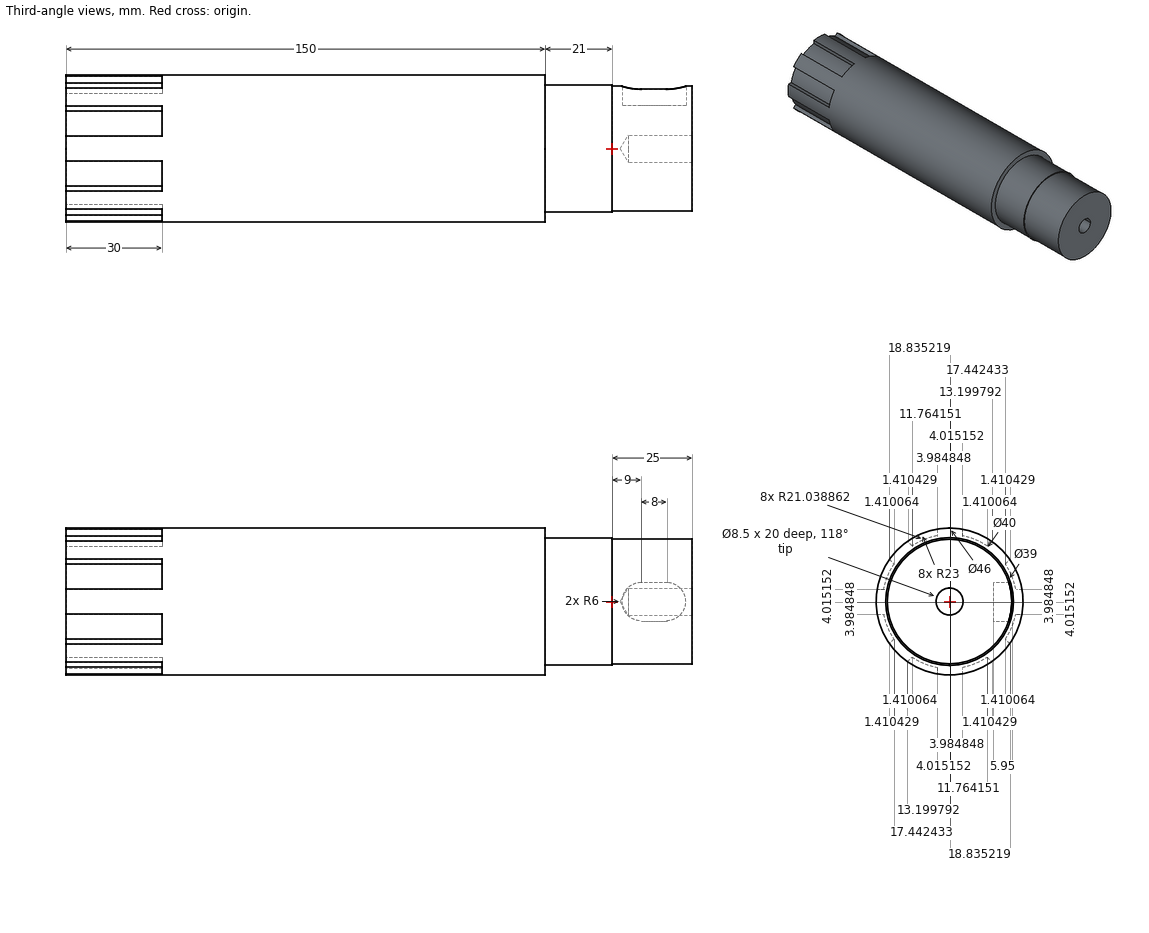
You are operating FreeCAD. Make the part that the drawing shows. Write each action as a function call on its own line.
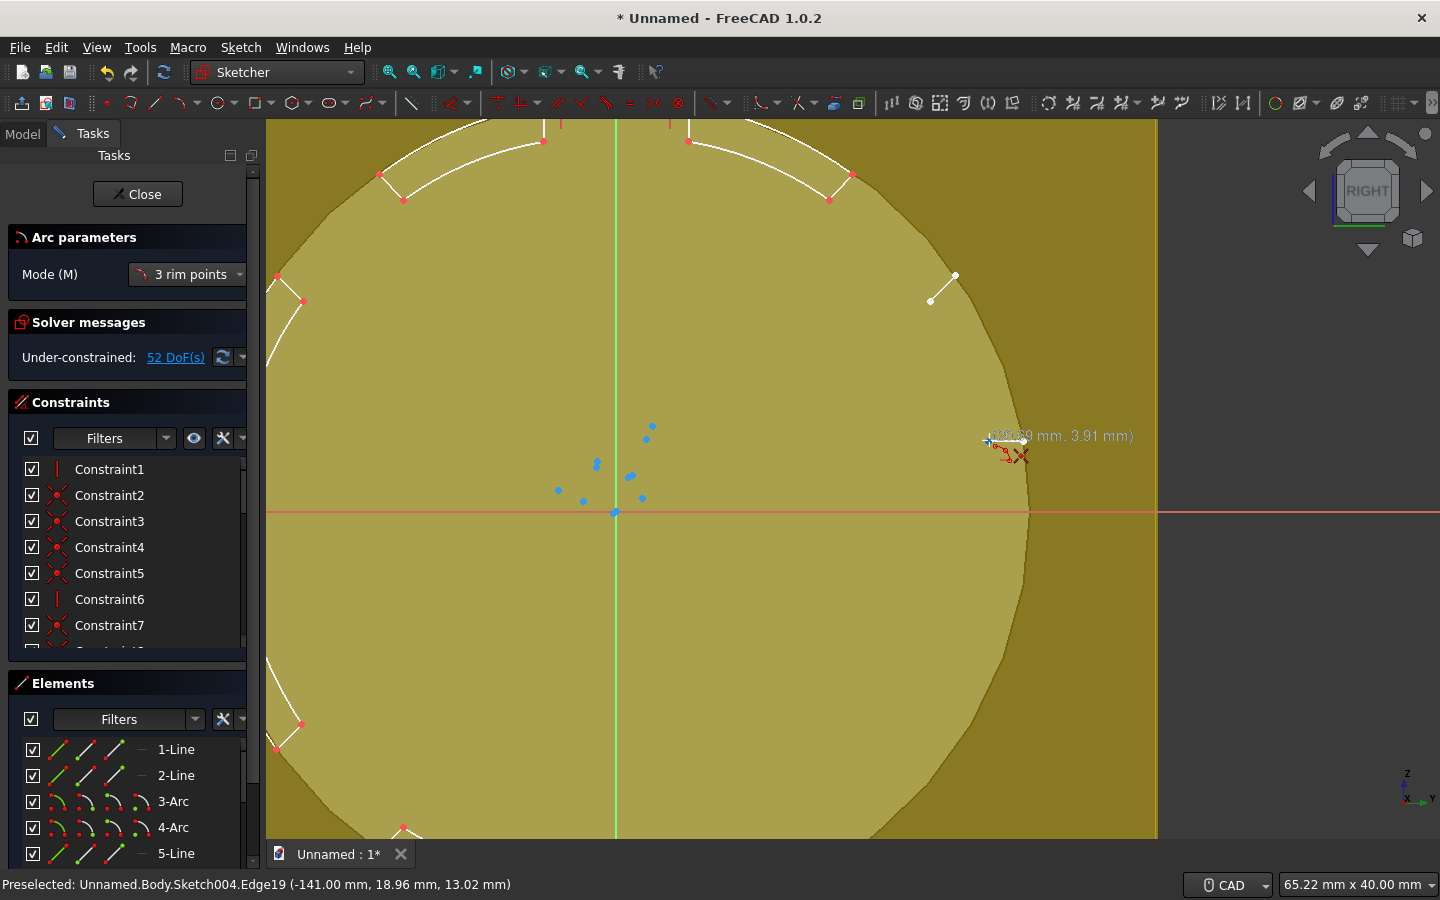
click(988, 441)
click(930, 301)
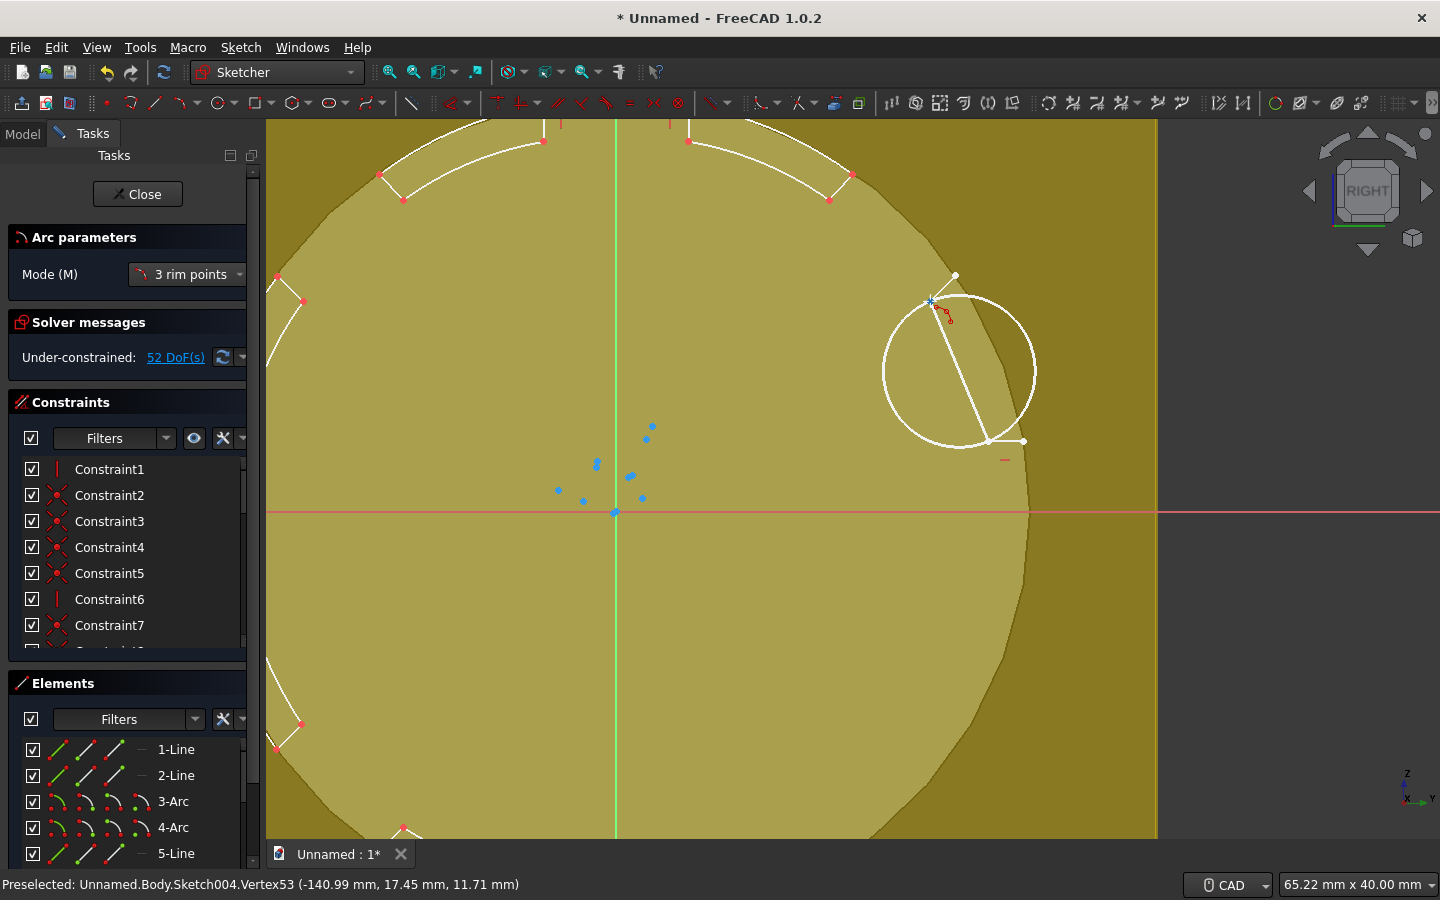
scroll(966, 367, up, 4)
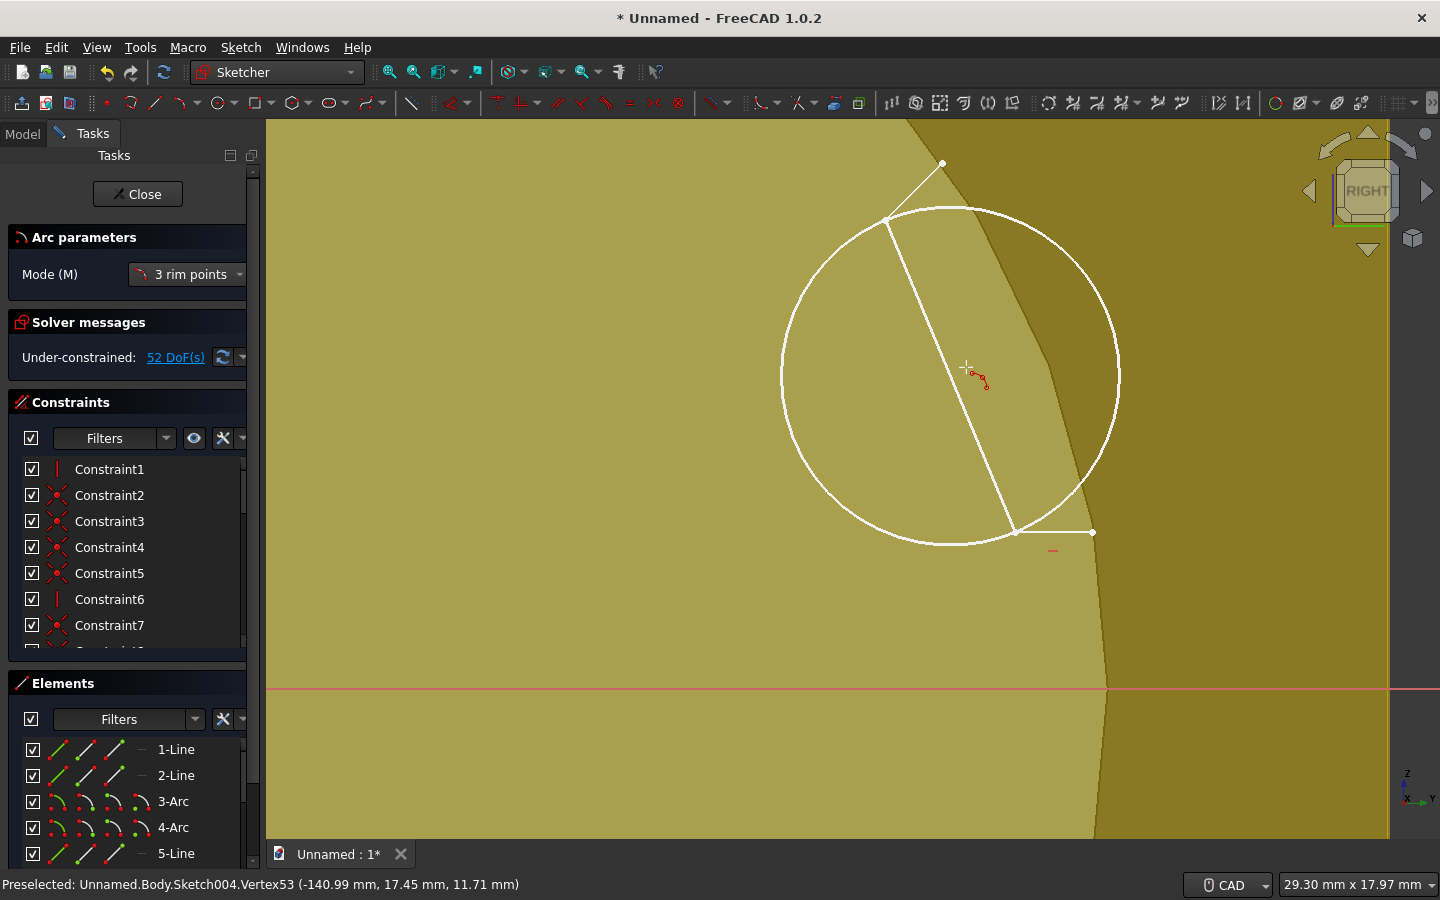
click(965, 367)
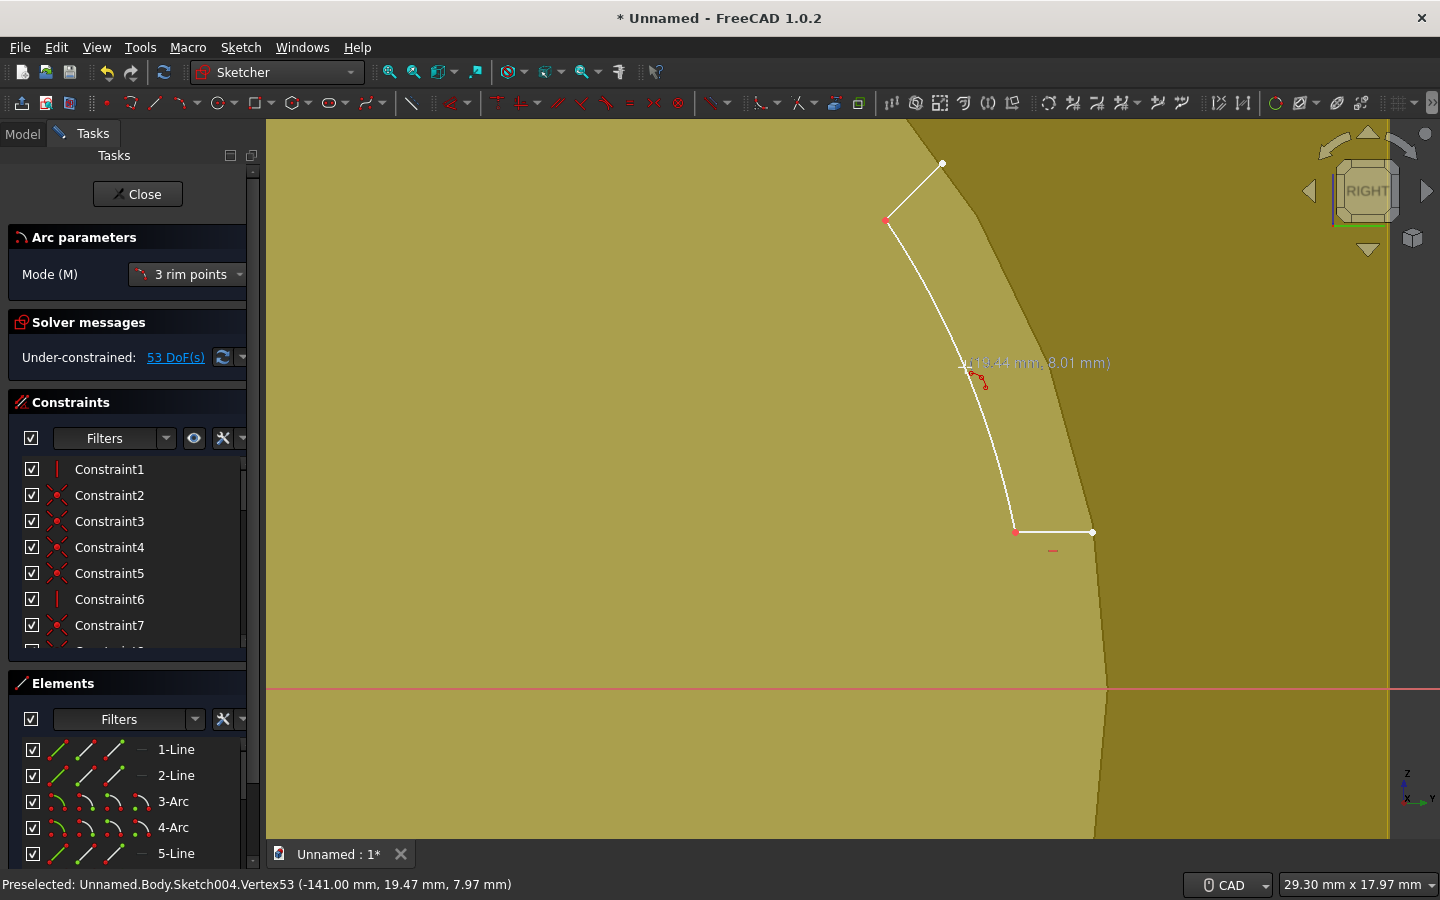
click(942, 163)
click(1092, 532)
click(1038, 337)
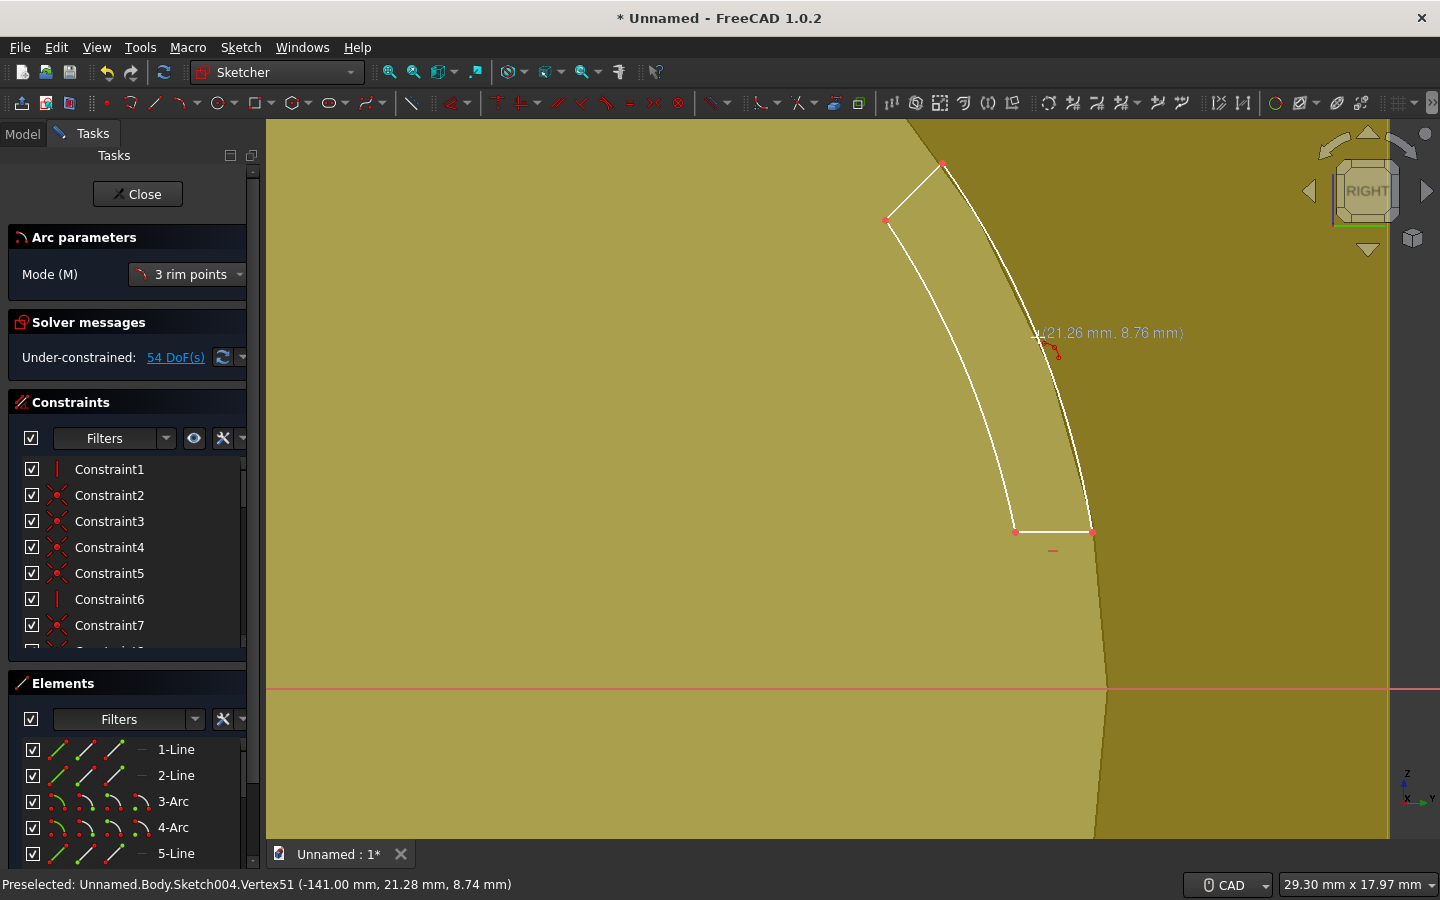
click(156, 104)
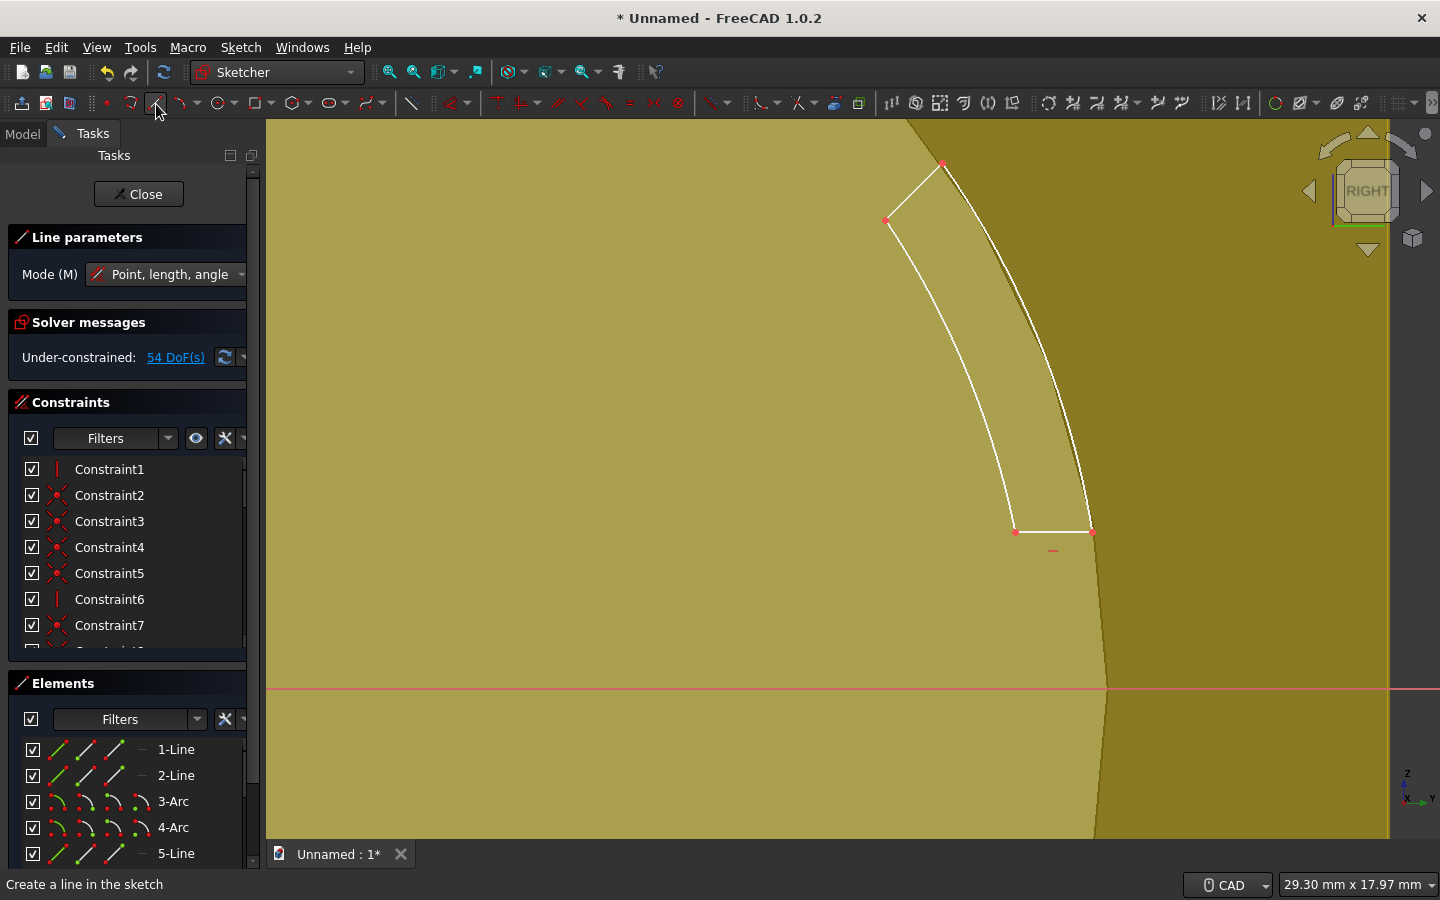
scroll(980, 410, down, 7)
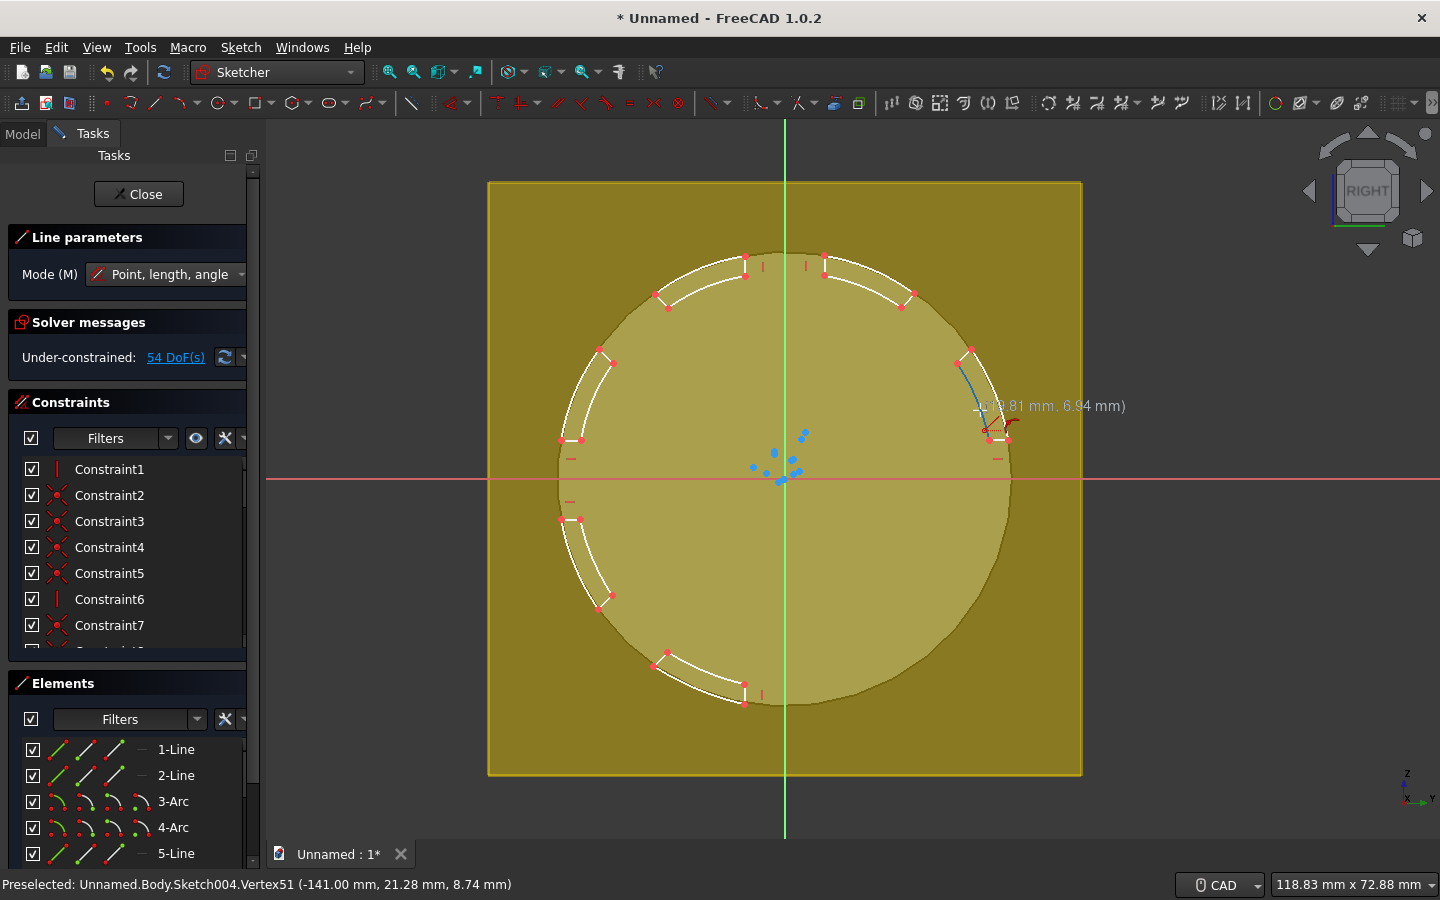
click(989, 519)
click(1008, 519)